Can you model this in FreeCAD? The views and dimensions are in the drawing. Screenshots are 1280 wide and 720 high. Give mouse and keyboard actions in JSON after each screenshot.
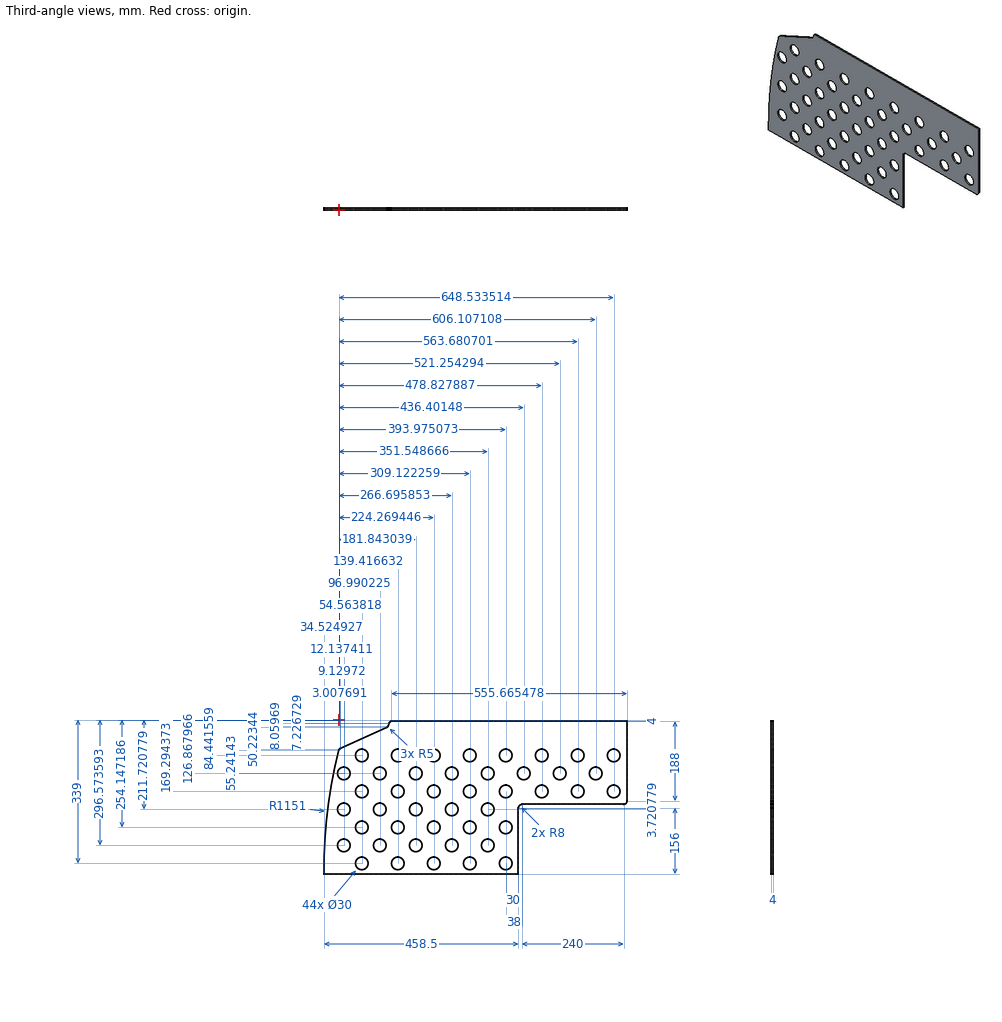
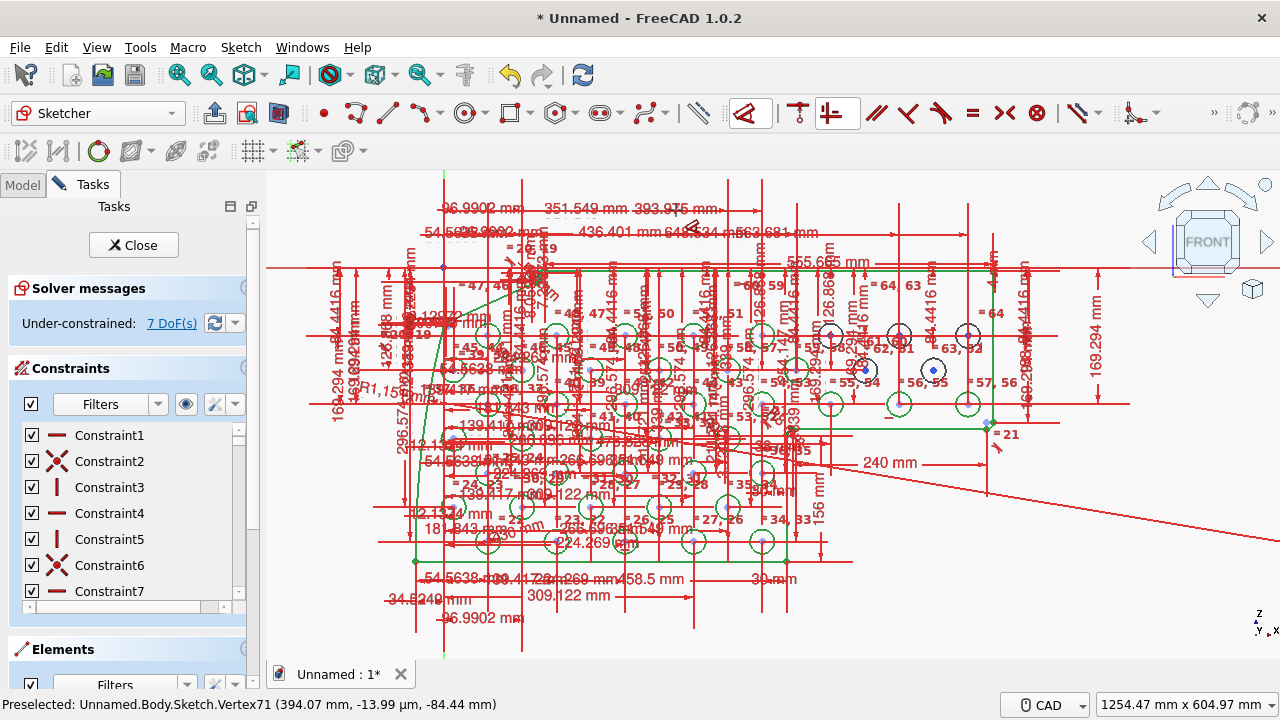
{"action": "left_click", "coordinate": [831, 336]}
{"action": "left_click", "coordinate": [773, 210]}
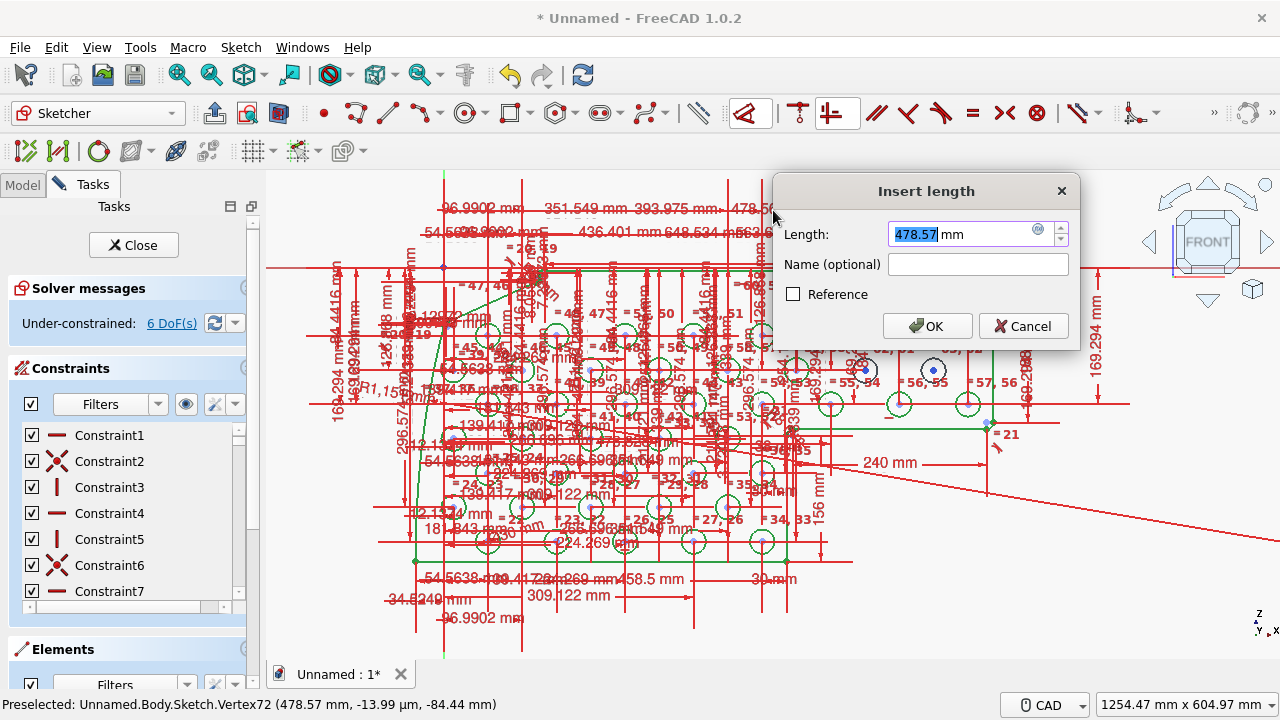
{"action": "type", "text": "478.827887"}
{"action": "key", "text": "Return"}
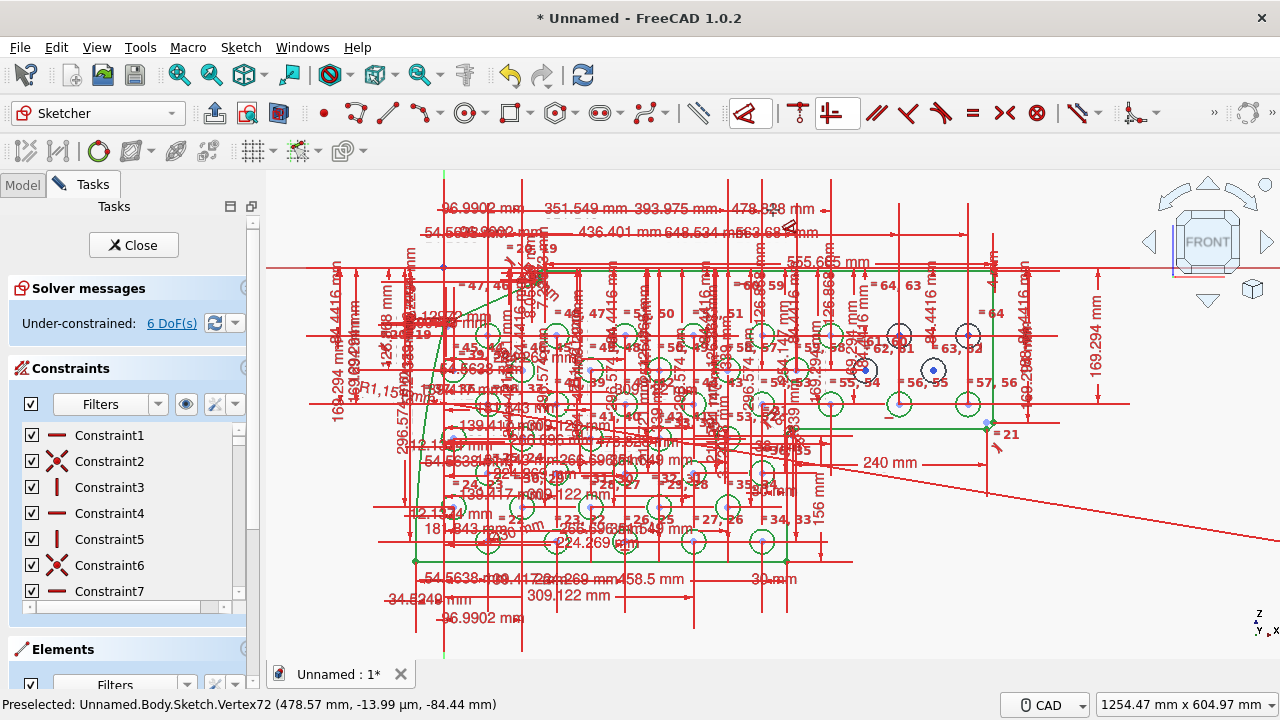
{"action": "left_click", "coordinate": [865, 371]}
{"action": "left_click", "coordinate": [802, 525]}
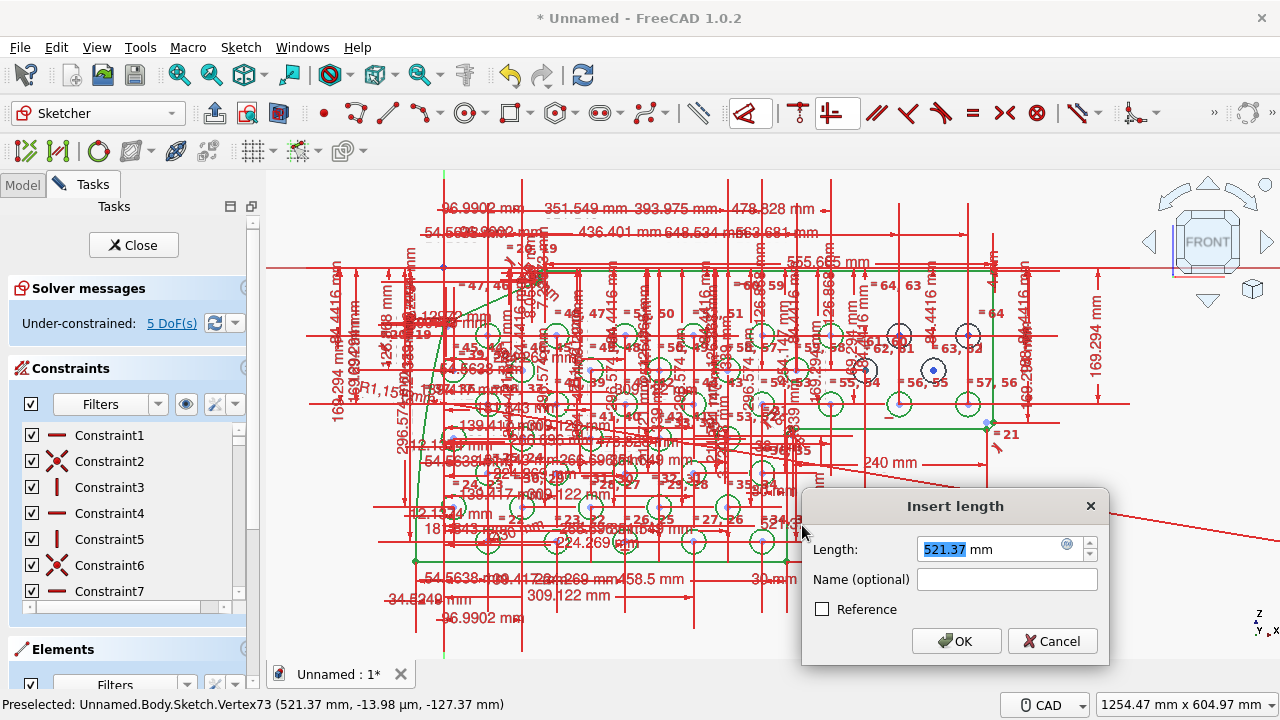
{"action": "type", "text": "521.254294"}
{"action": "key", "text": "Return"}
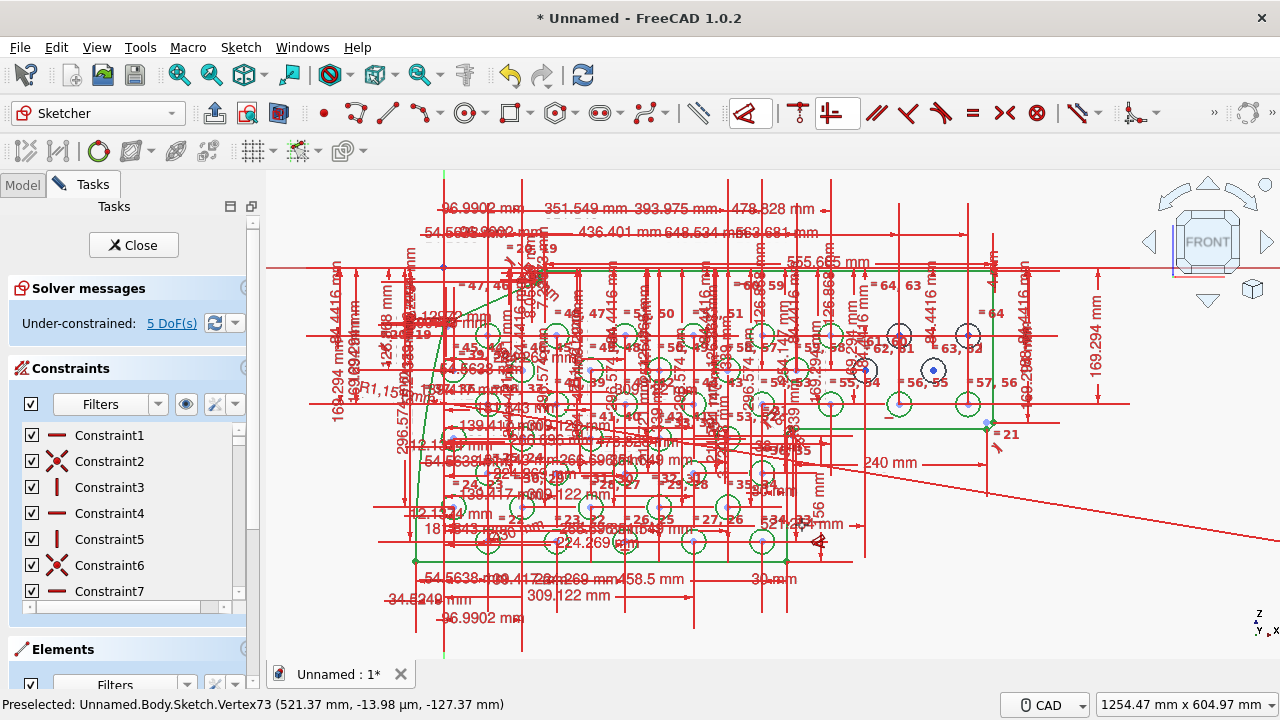
{"action": "left_click", "coordinate": [865, 371]}
{"action": "left_click", "coordinate": [899, 283]}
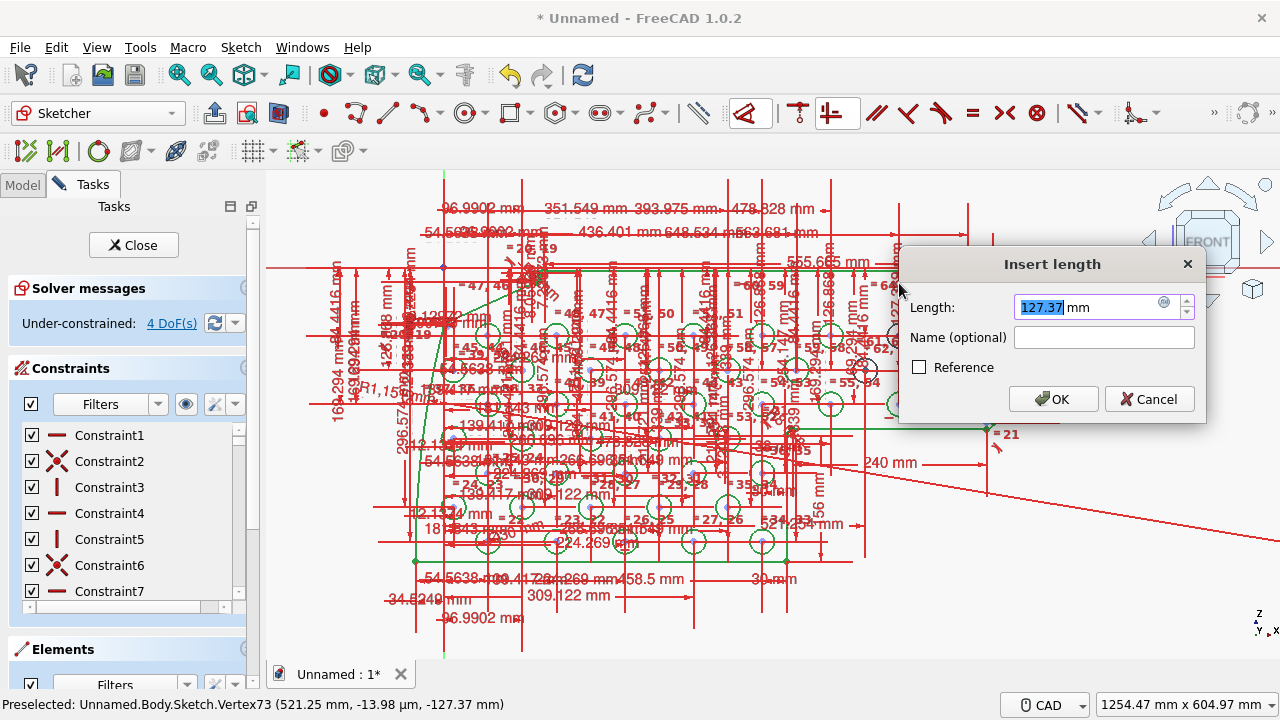
{"action": "type", "text": "126.867966"}
{"action": "key", "text": "Return"}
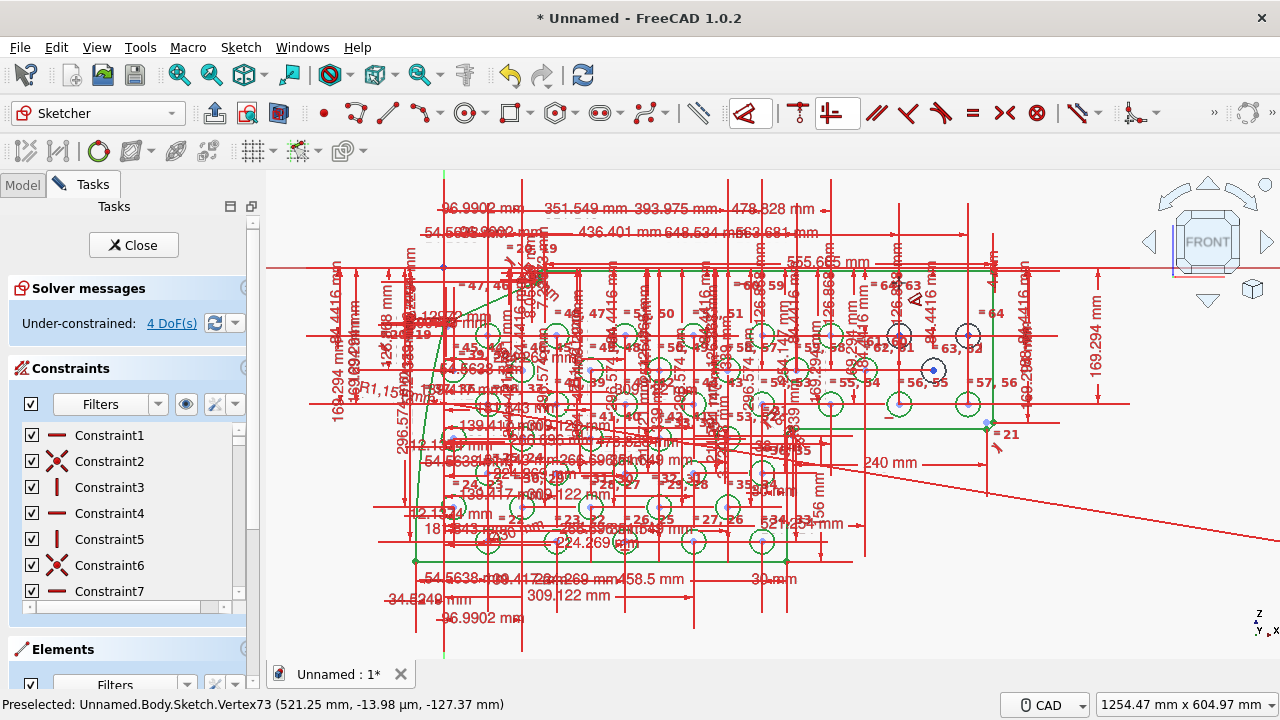
{"action": "left_click", "coordinate": [934, 371]}
{"action": "left_click", "coordinate": [860, 234]}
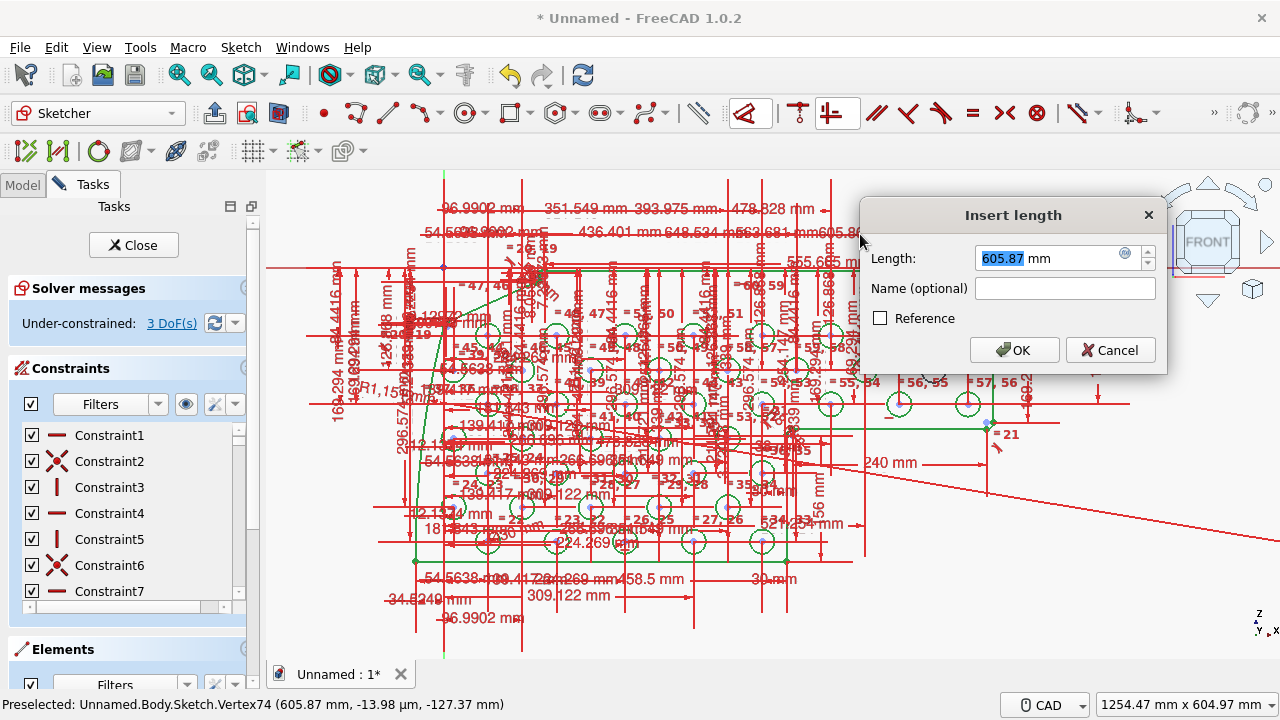
{"action": "type", "text": "606.107108"}
{"action": "key", "text": "Return"}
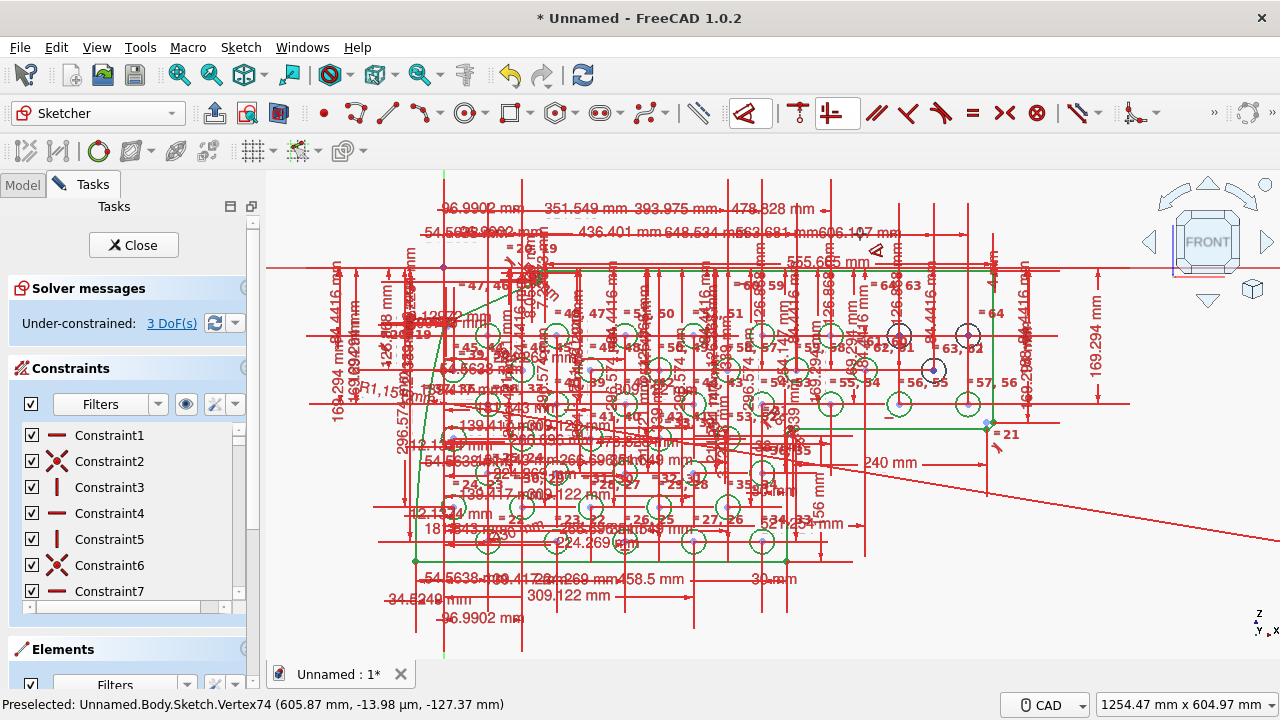
{"action": "left_click", "coordinate": [934, 371]}
{"action": "left_click", "coordinate": [1114, 295]}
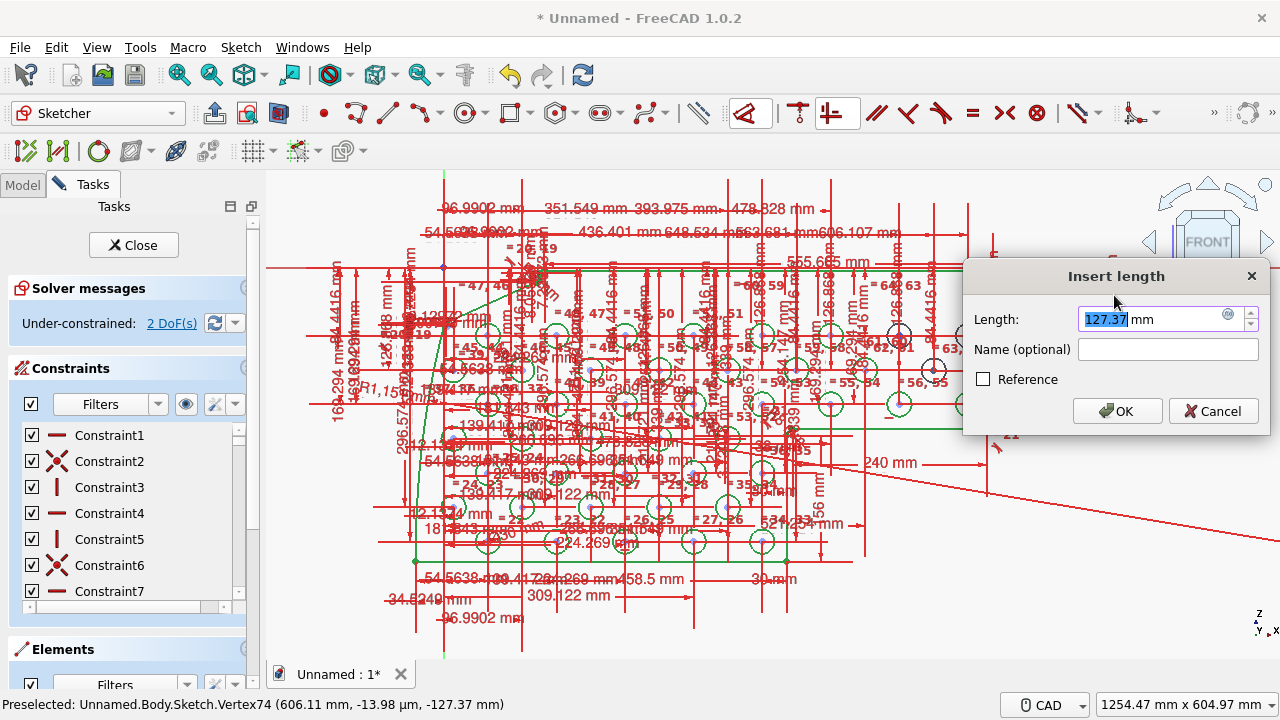
{"action": "type", "text": "126.867966"}
{"action": "key", "text": "Return"}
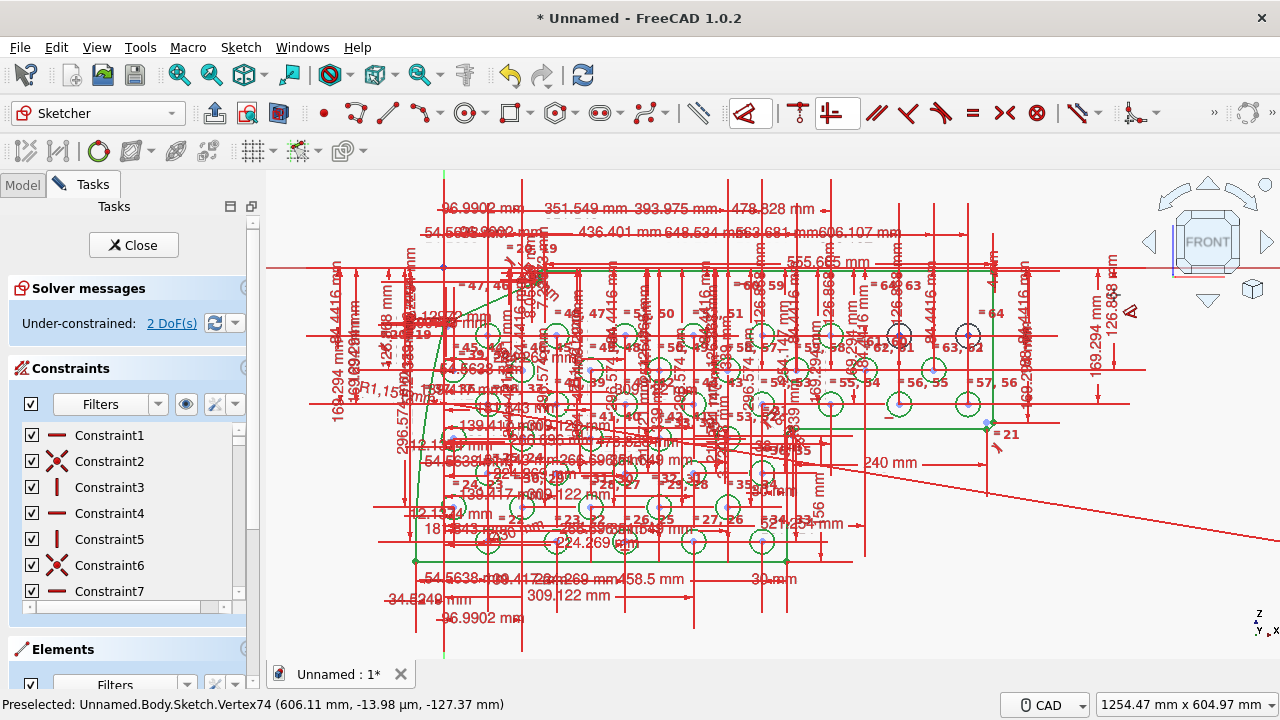
{"action": "left_click", "coordinate": [899, 336]}
{"action": "left_click", "coordinate": [567, 234]}